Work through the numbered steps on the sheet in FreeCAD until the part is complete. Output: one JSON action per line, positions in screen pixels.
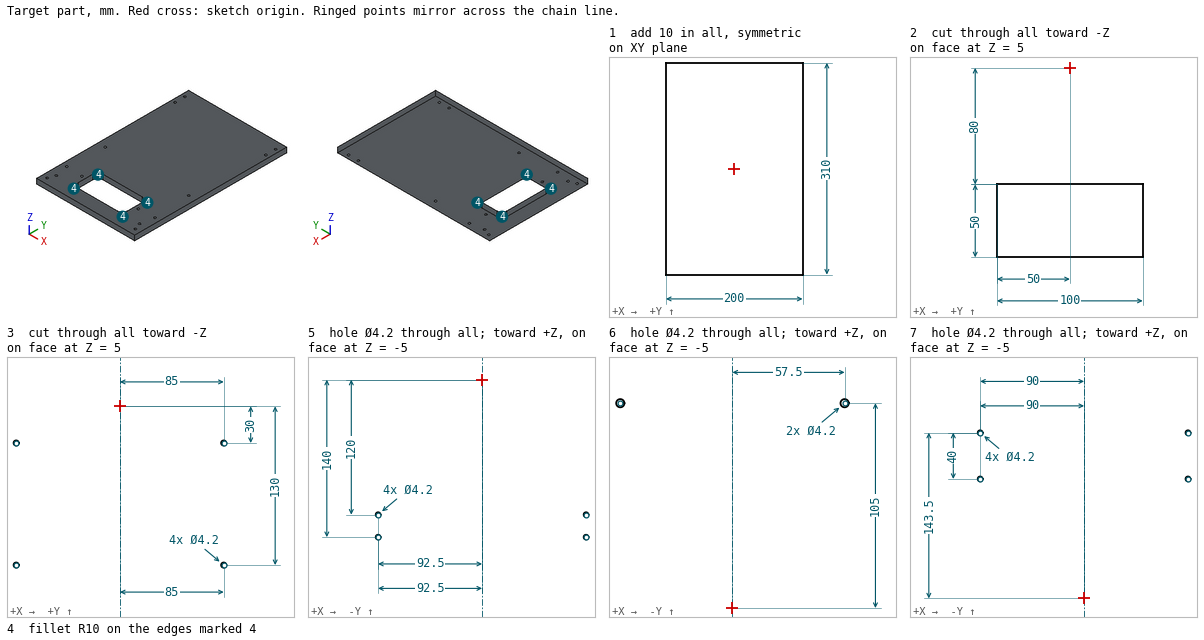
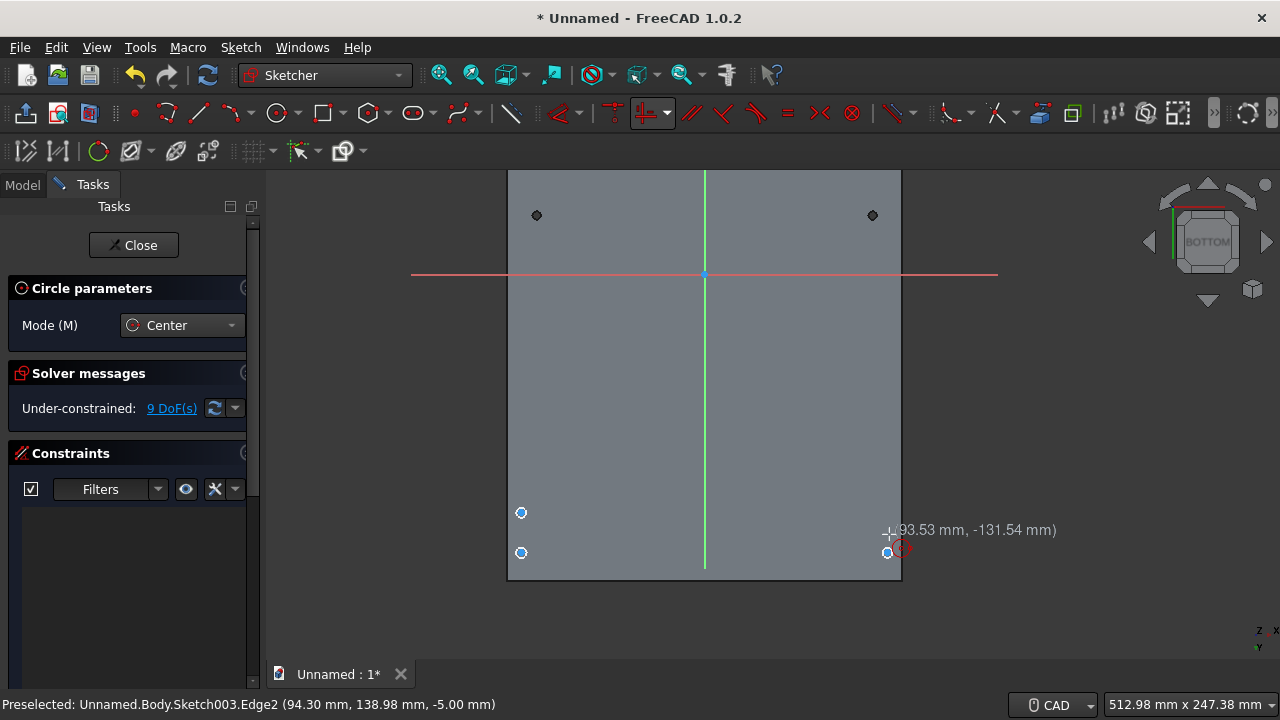
{"action": "left_click", "coordinate": [887, 512]}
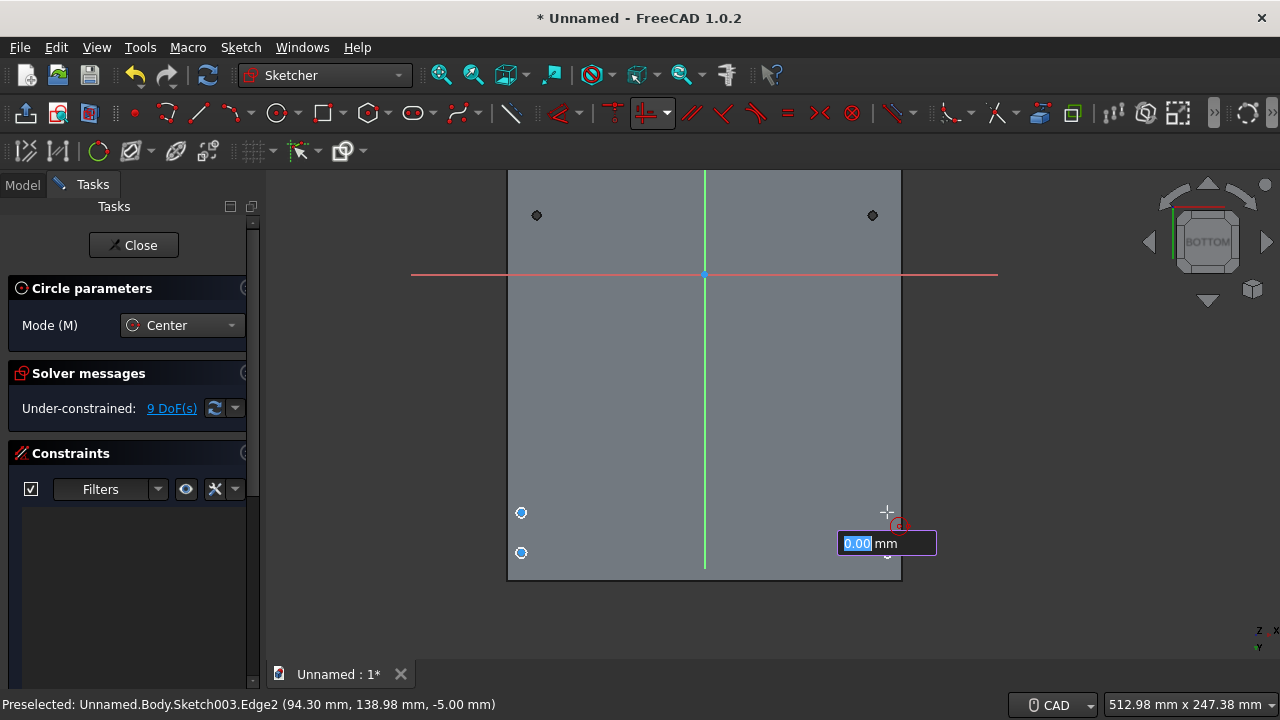
{"action": "scroll", "coordinate": [890, 509], "scroll_direction": "up", "scroll_amount": 7}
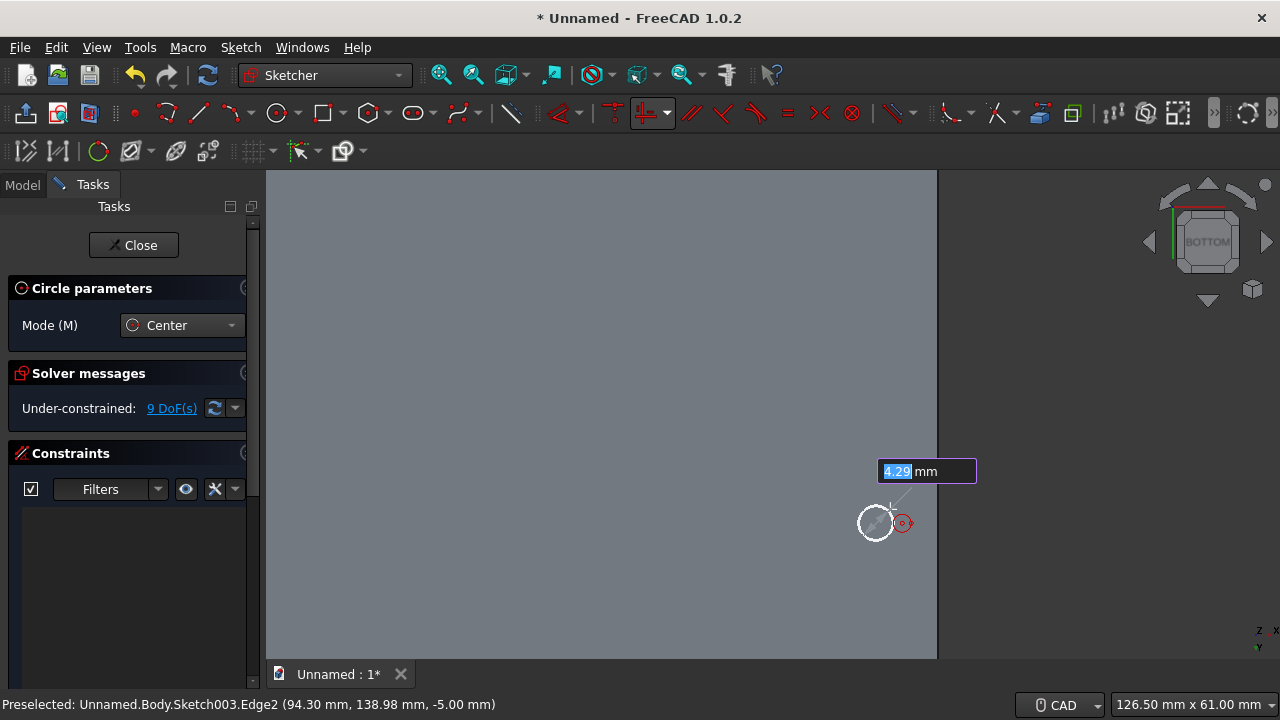
{"action": "left_click", "coordinate": [890, 507]}
{"action": "key", "text": "Escape"}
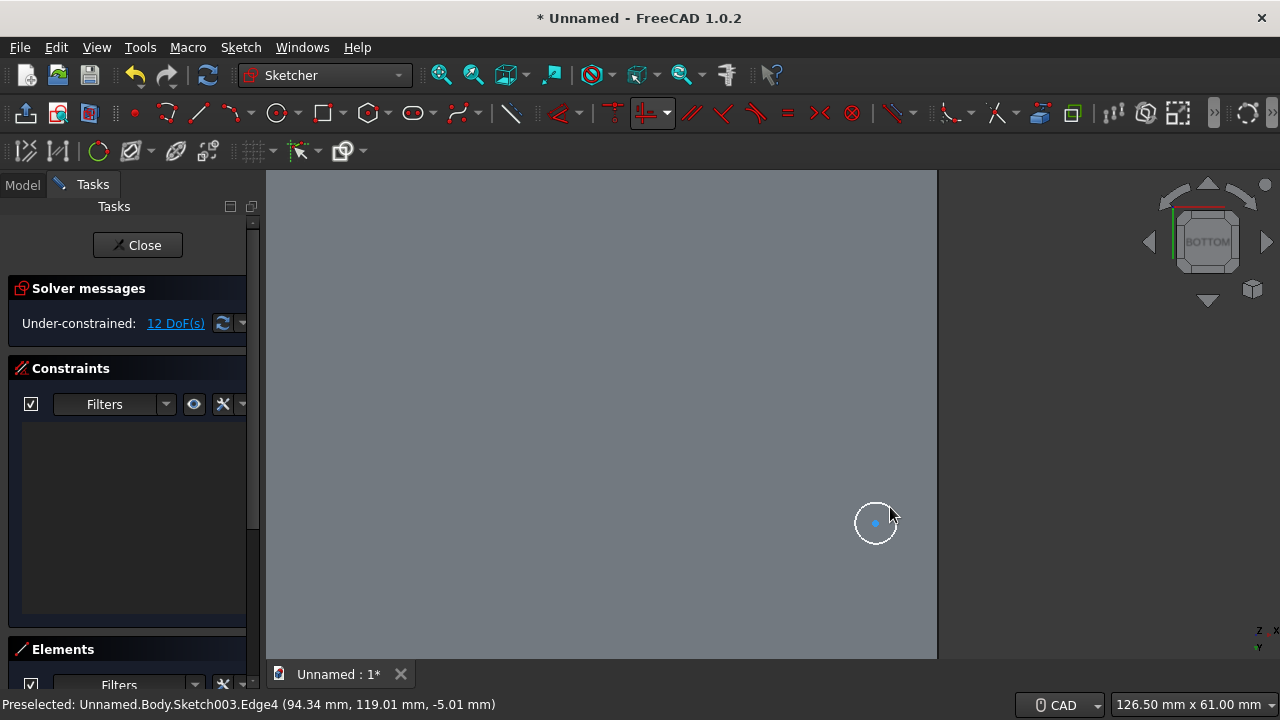
{"action": "scroll", "coordinate": [890, 509], "scroll_direction": "down", "scroll_amount": 7}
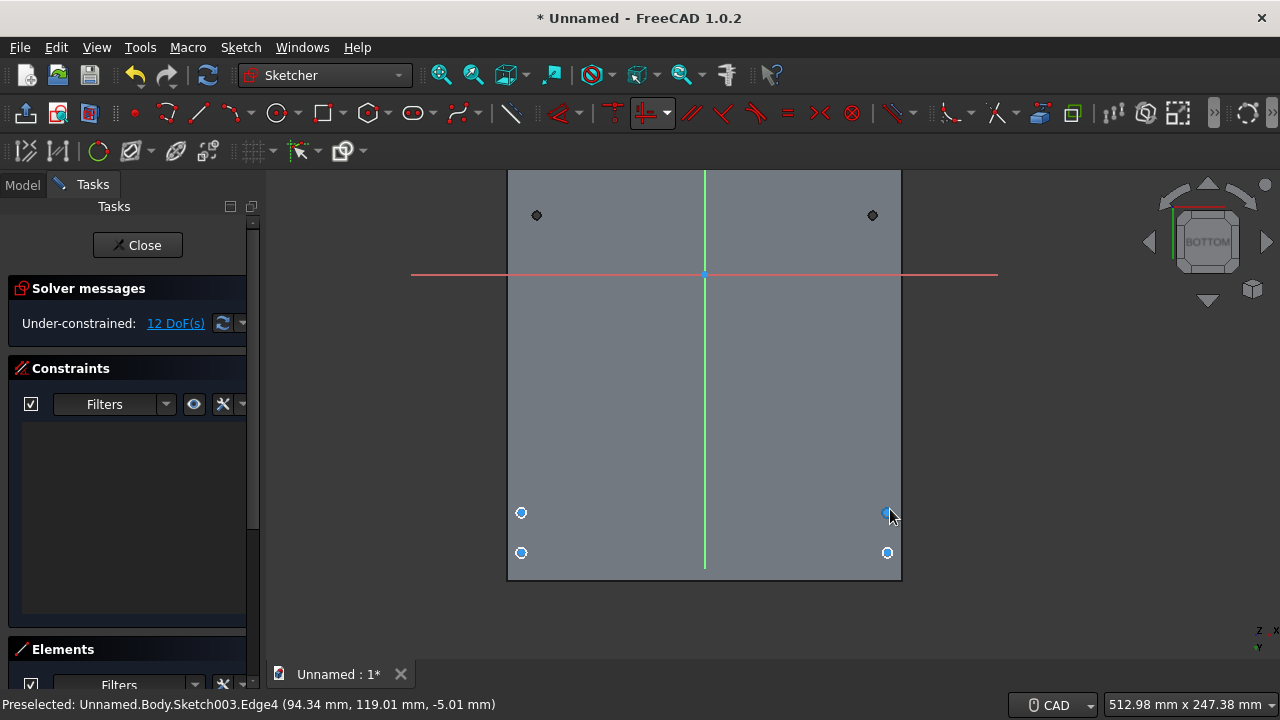
{"action": "scroll", "coordinate": [525, 509], "scroll_direction": "up", "scroll_amount": 6}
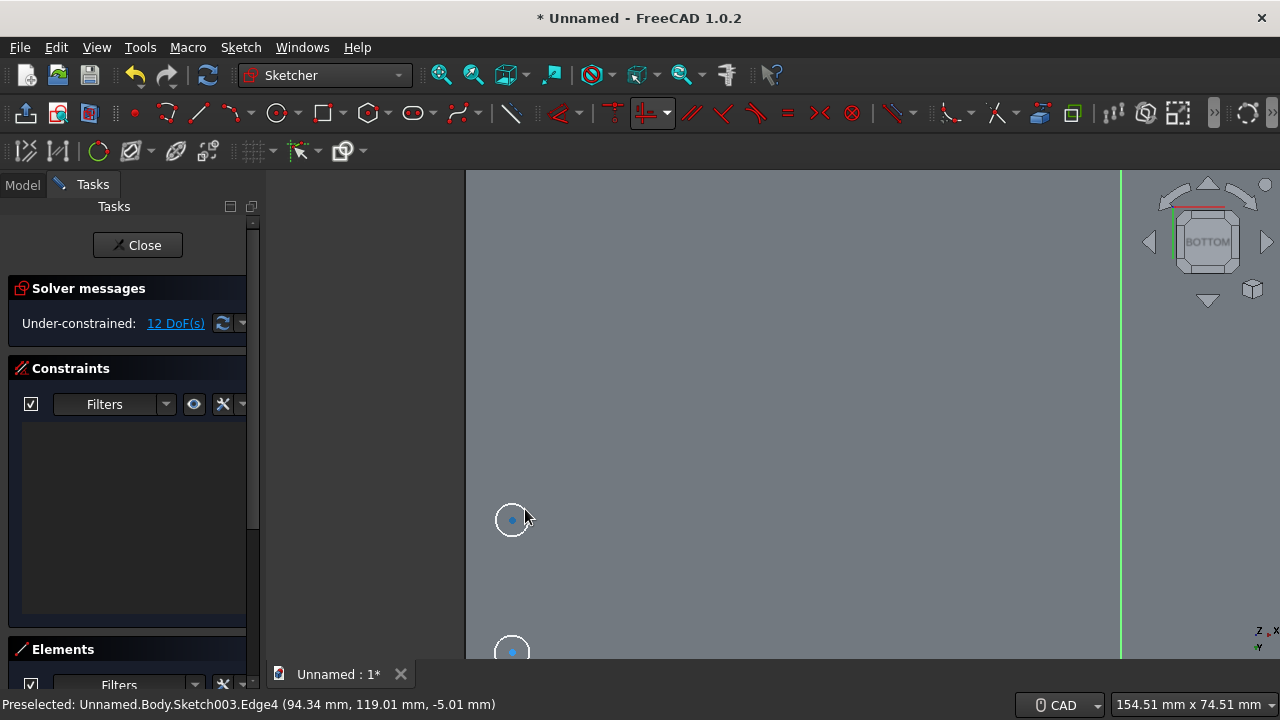
{"action": "left_click", "coordinate": [524, 509]}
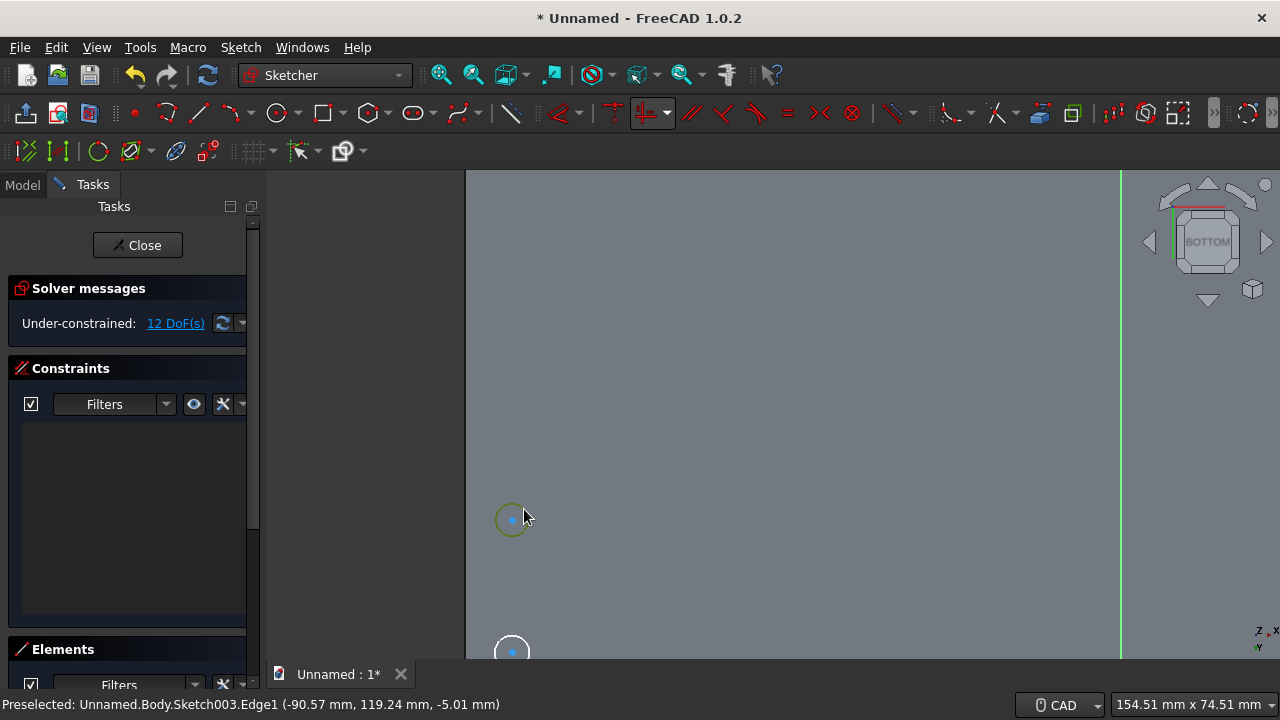
{"action": "scroll", "coordinate": [525, 509], "scroll_direction": "down", "scroll_amount": 6}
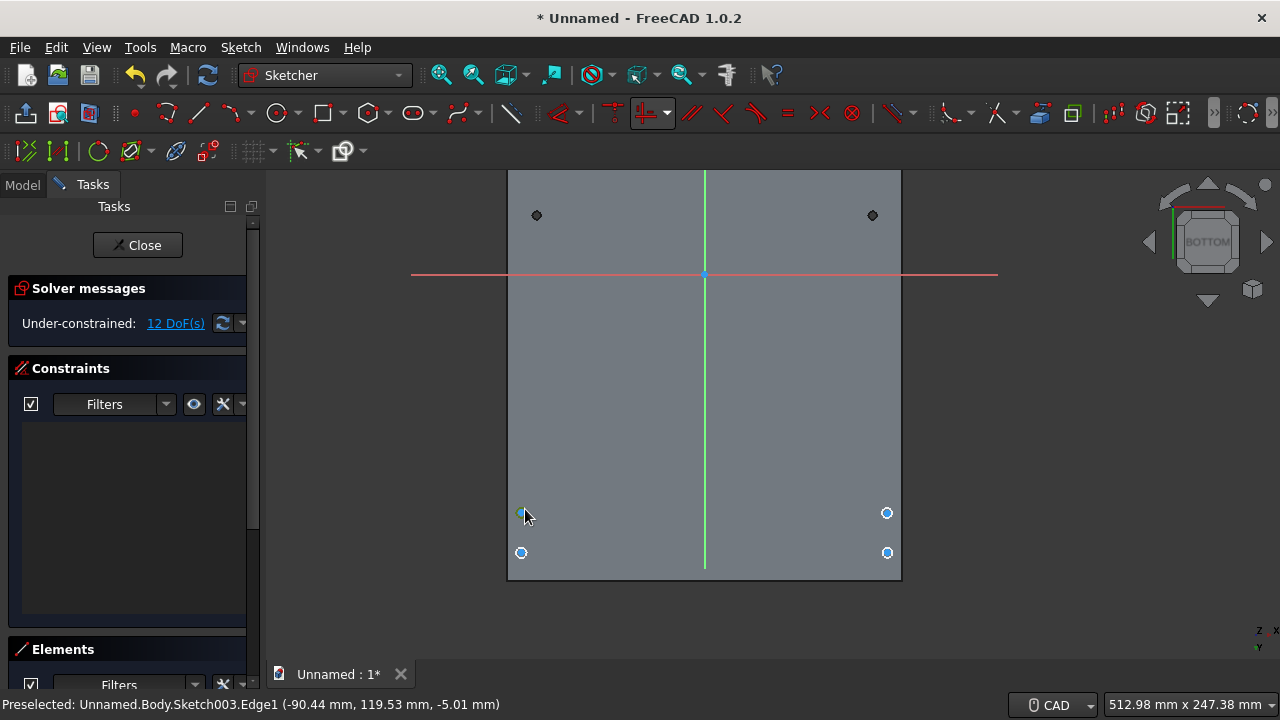
{"action": "scroll", "coordinate": [525, 549], "scroll_direction": "up", "scroll_amount": 5}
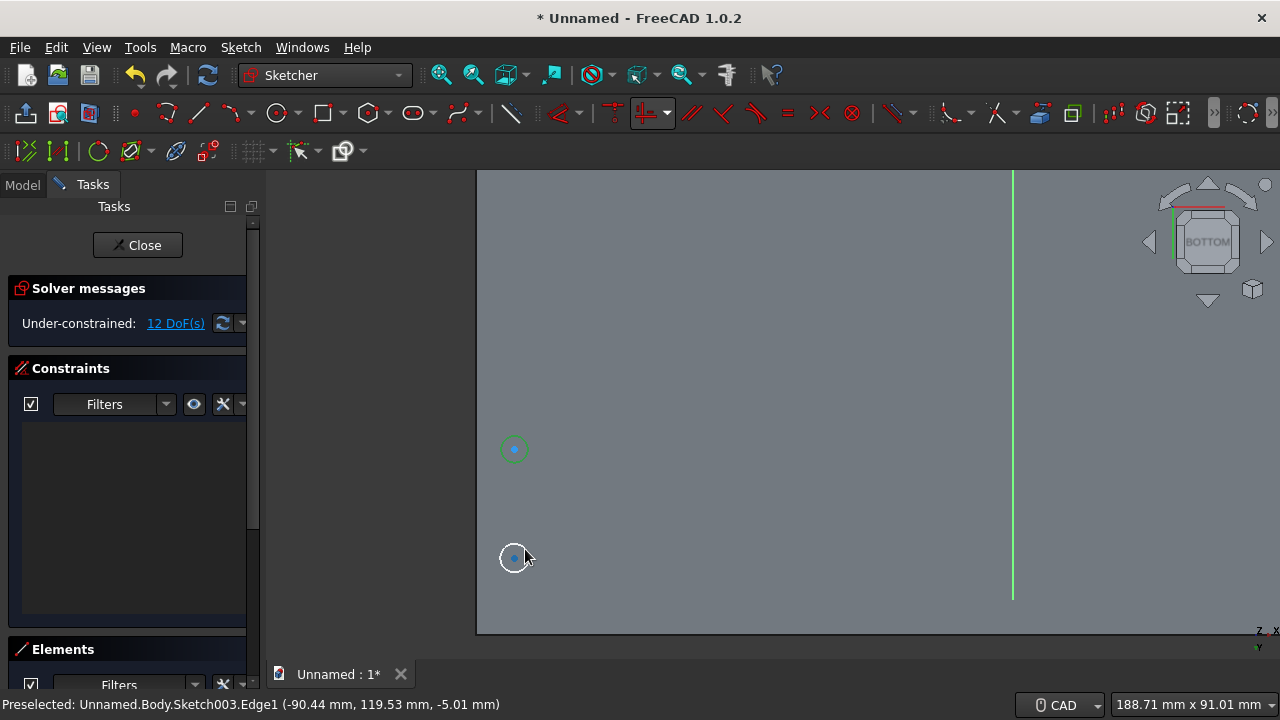
{"action": "left_click", "coordinate": [524, 548]}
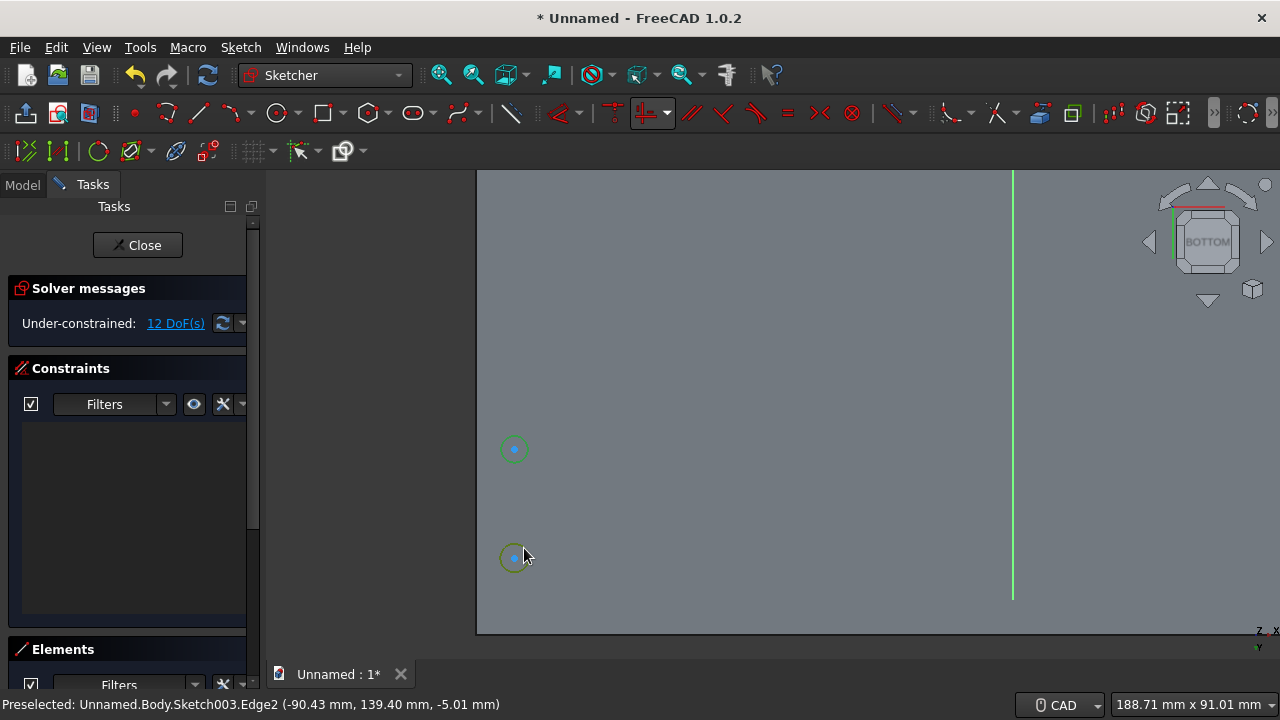
{"action": "scroll", "coordinate": [525, 549], "scroll_direction": "down", "scroll_amount": 5}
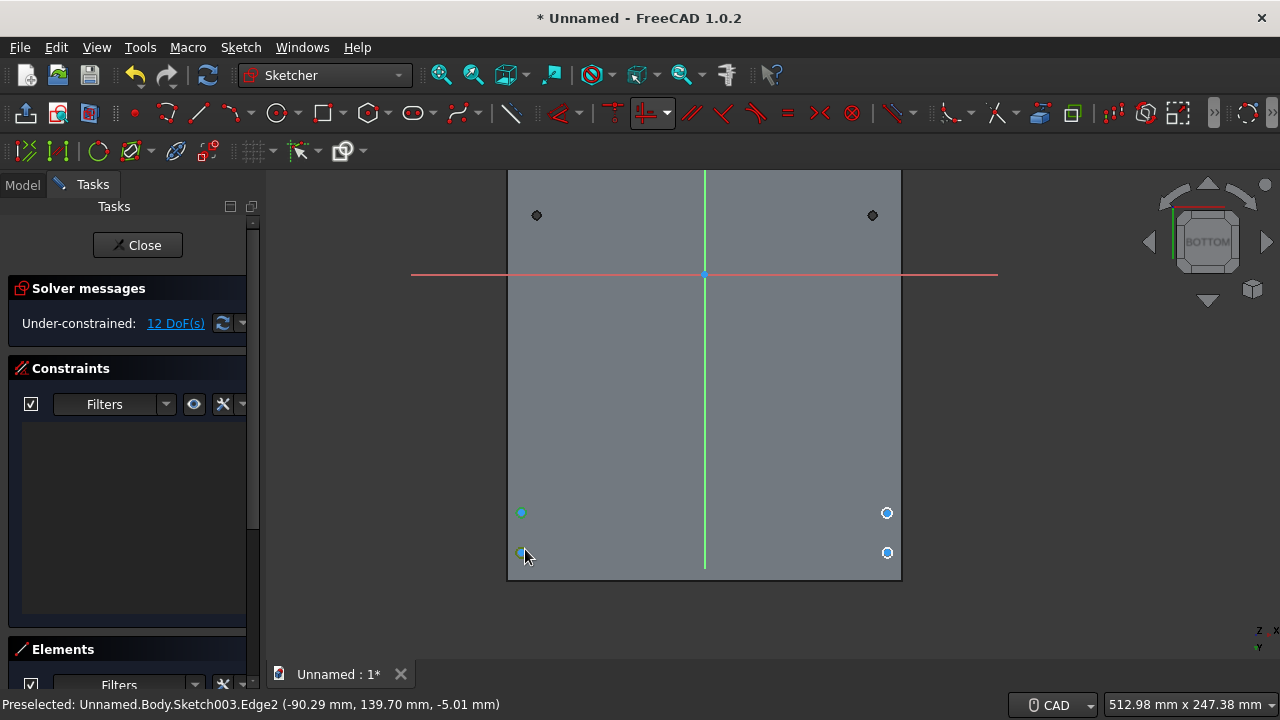
{"action": "scroll", "coordinate": [891, 549], "scroll_direction": "up", "scroll_amount": 6}